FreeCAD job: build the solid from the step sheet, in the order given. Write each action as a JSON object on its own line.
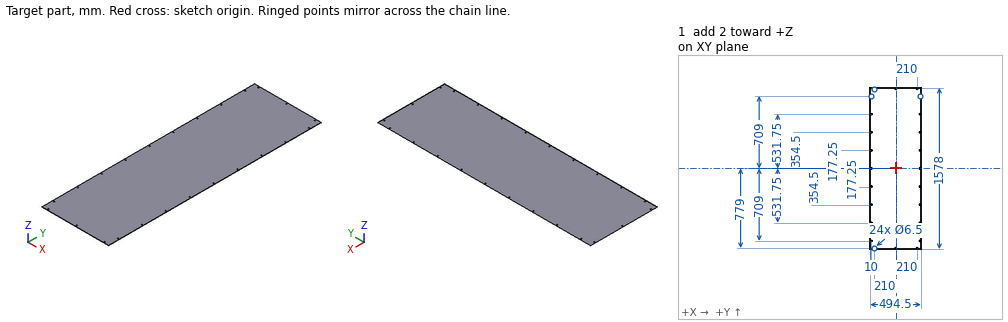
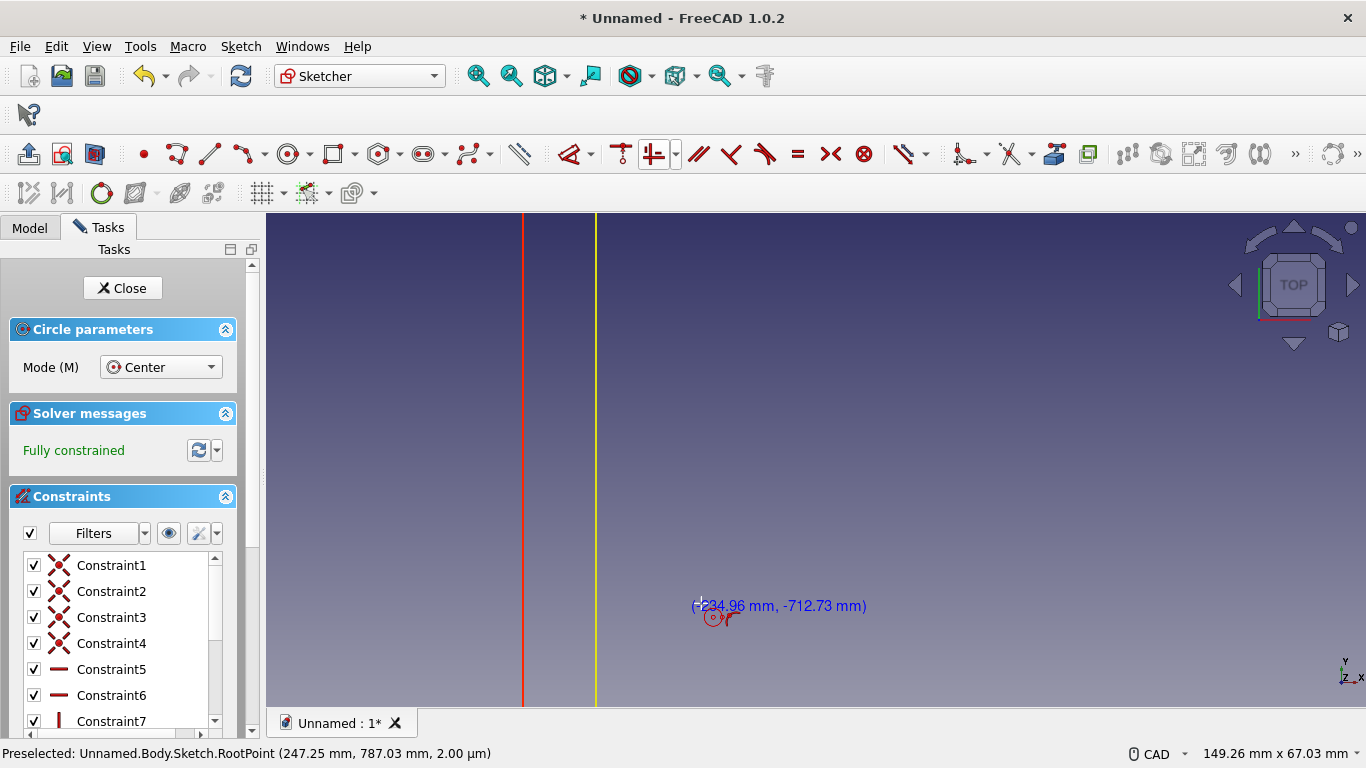
{"action": "scroll", "coordinate": [701, 603], "scroll_direction": "down", "scroll_amount": 18}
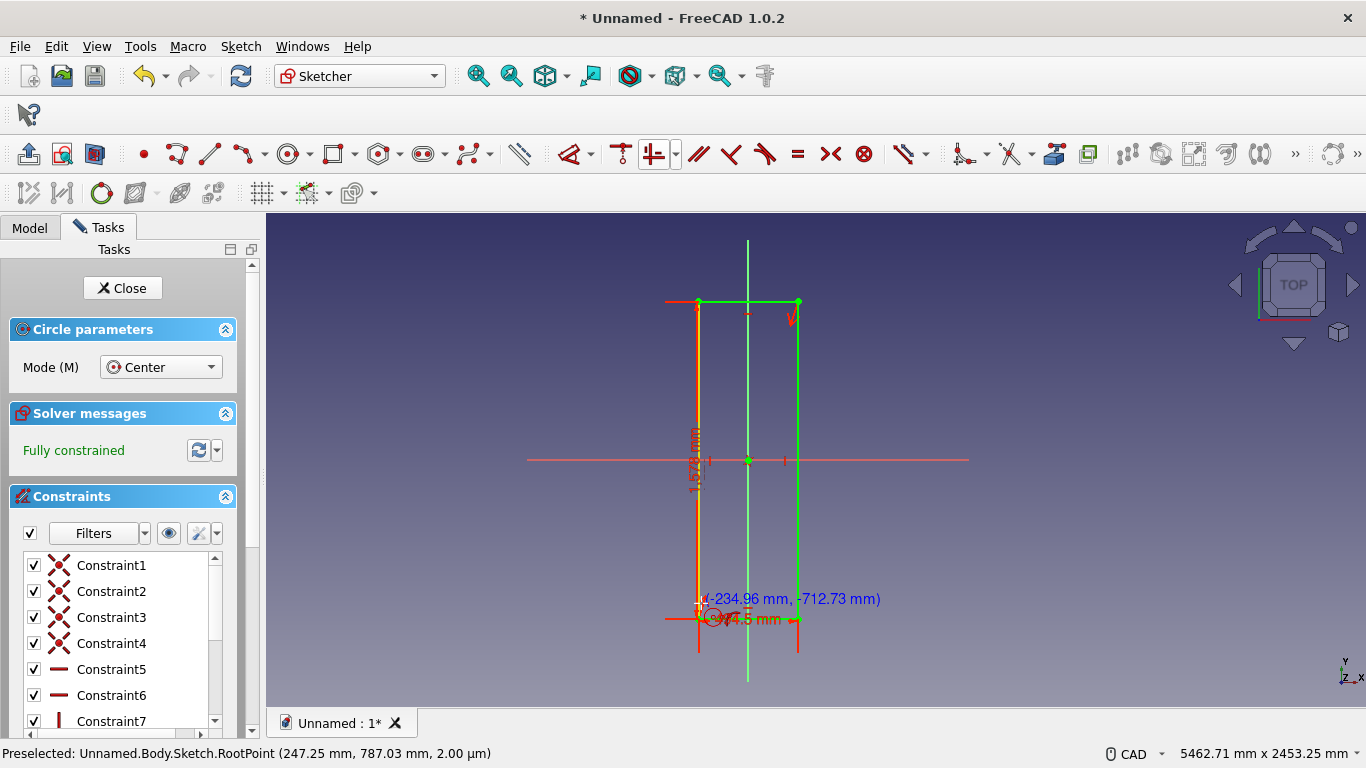
{"action": "scroll", "coordinate": [701, 603], "scroll_direction": "up", "scroll_amount": 11}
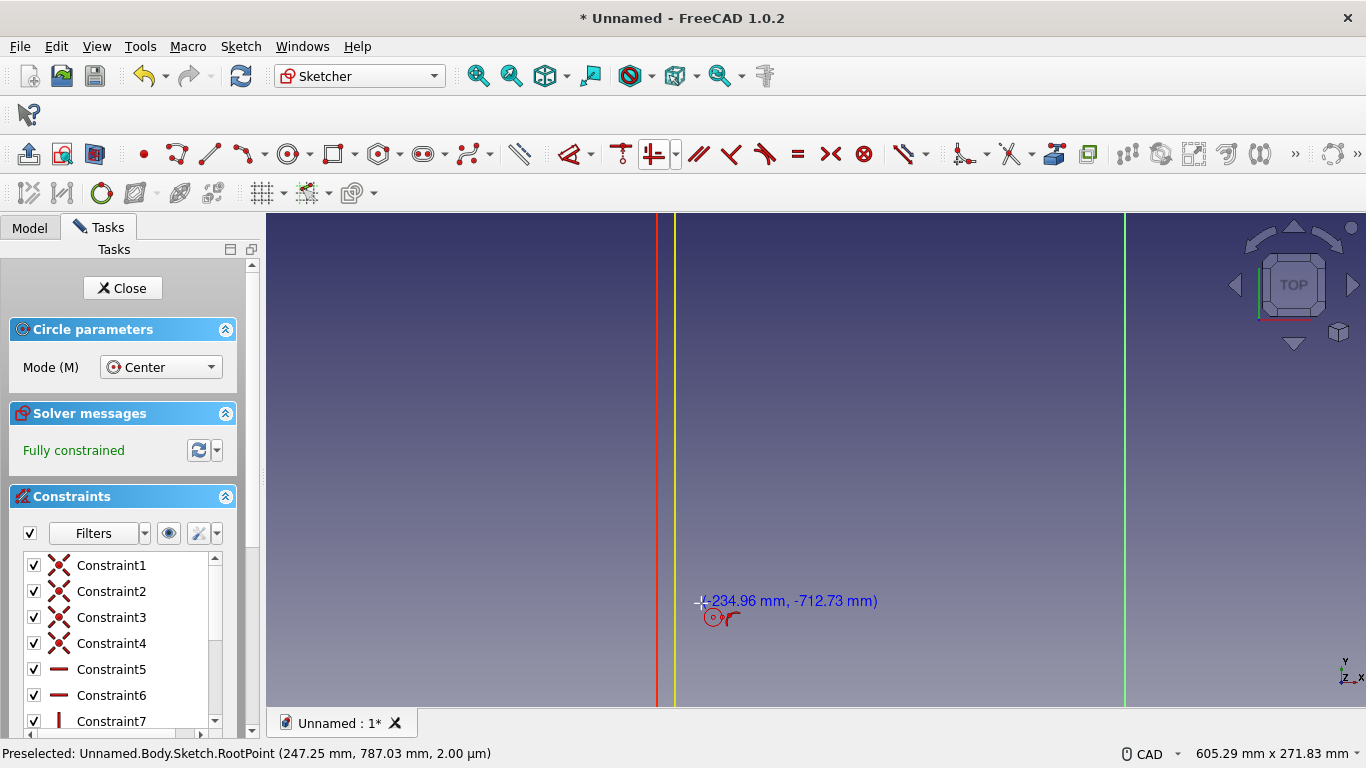
{"action": "left_click", "coordinate": [694, 599]}
{"action": "mouse_move", "coordinate": [698, 595]}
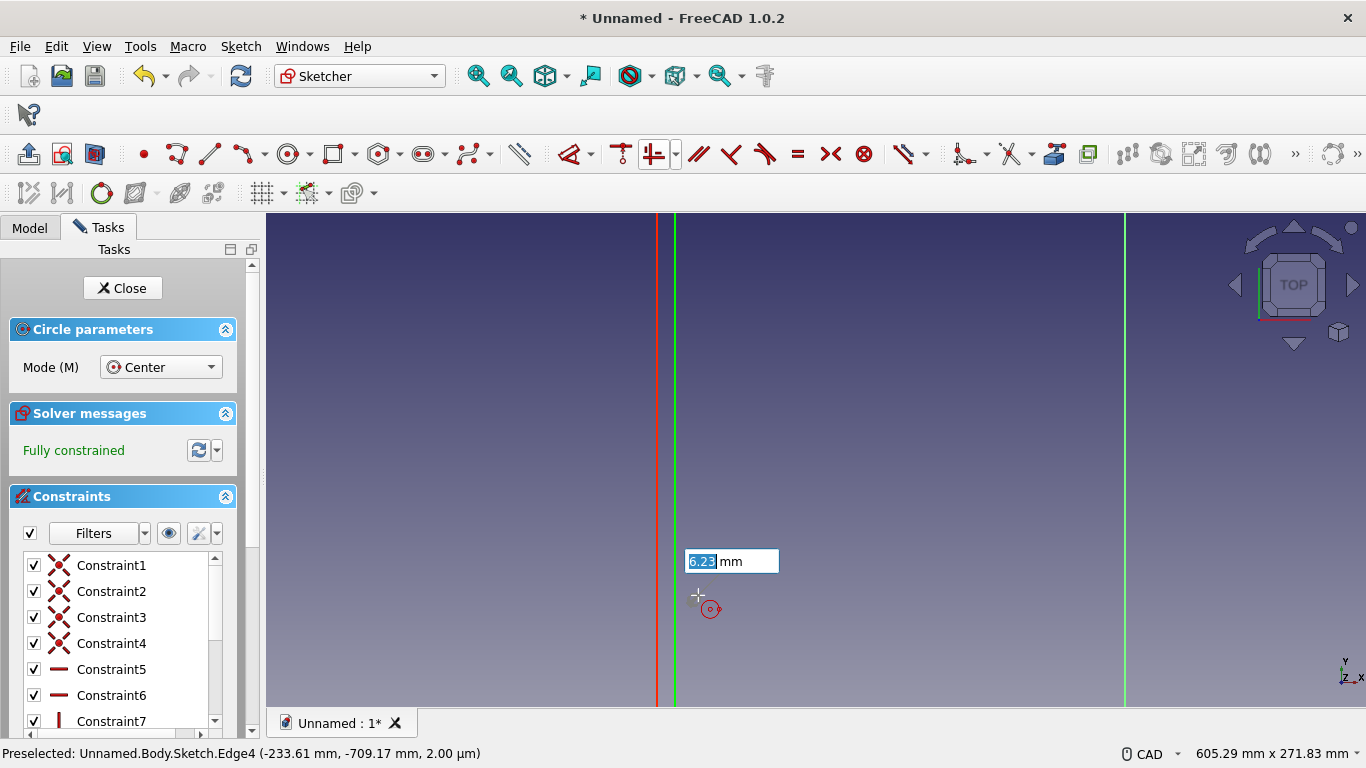
{"action": "type", "text": "6.5"}
{"action": "key", "text": "Return"}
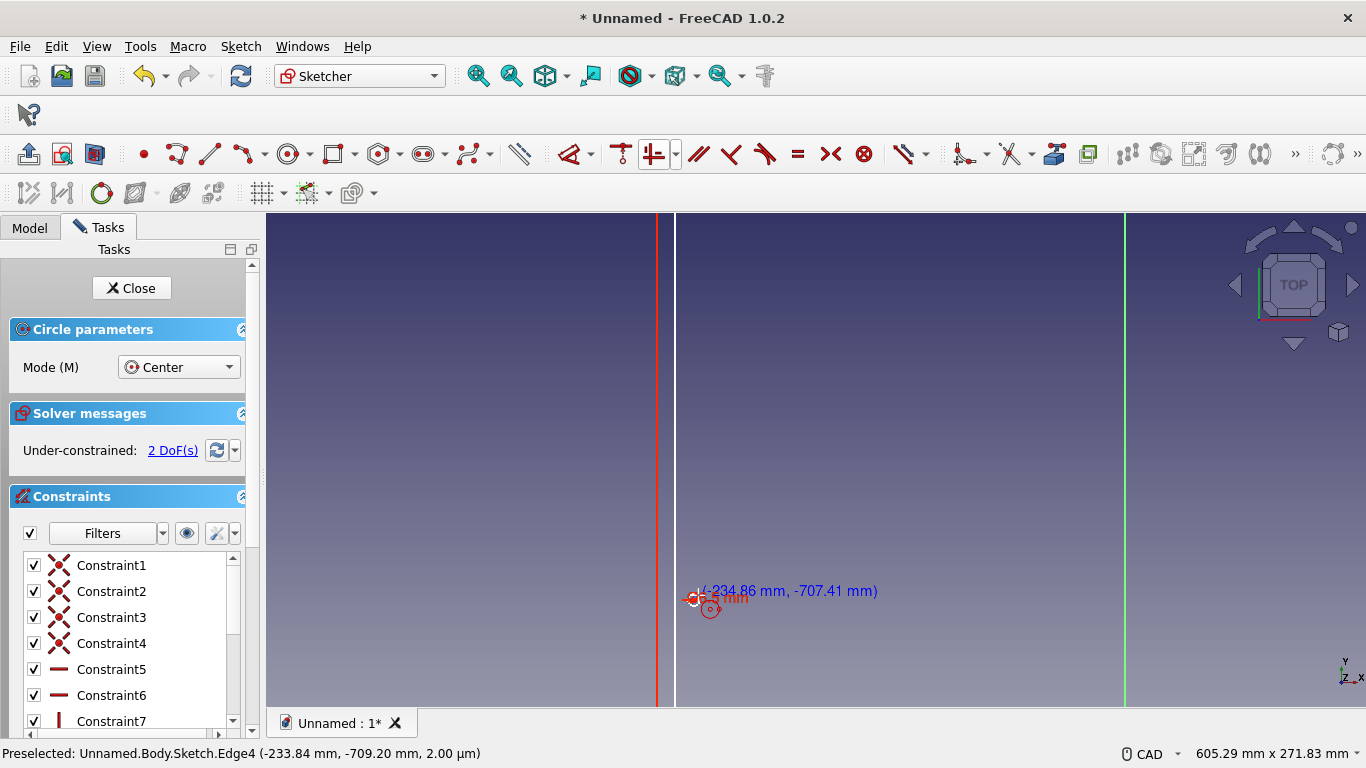
{"action": "scroll", "coordinate": [700, 603], "scroll_direction": "down", "scroll_amount": 11}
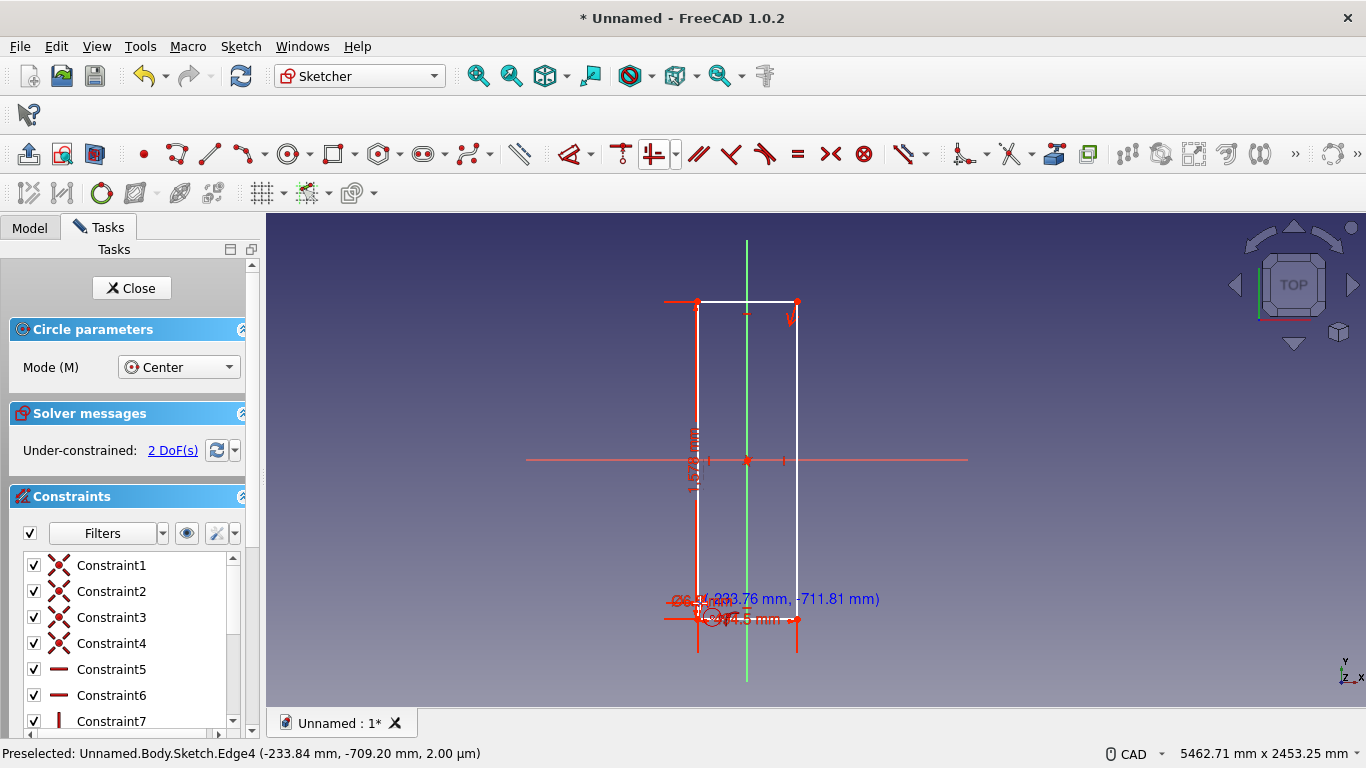
{"action": "scroll", "coordinate": [705, 617], "scroll_direction": "up", "scroll_amount": 18}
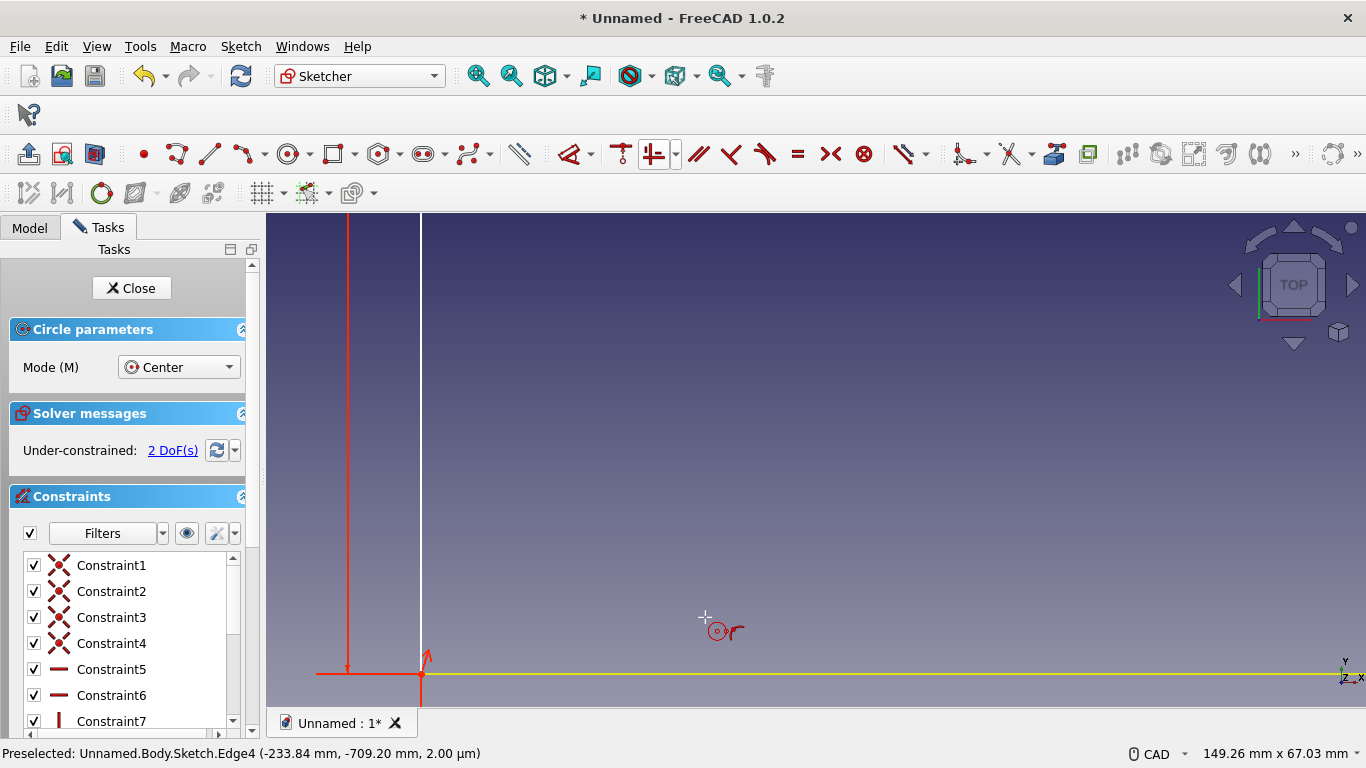
{"action": "scroll", "coordinate": [705, 617], "scroll_direction": "down", "scroll_amount": 18}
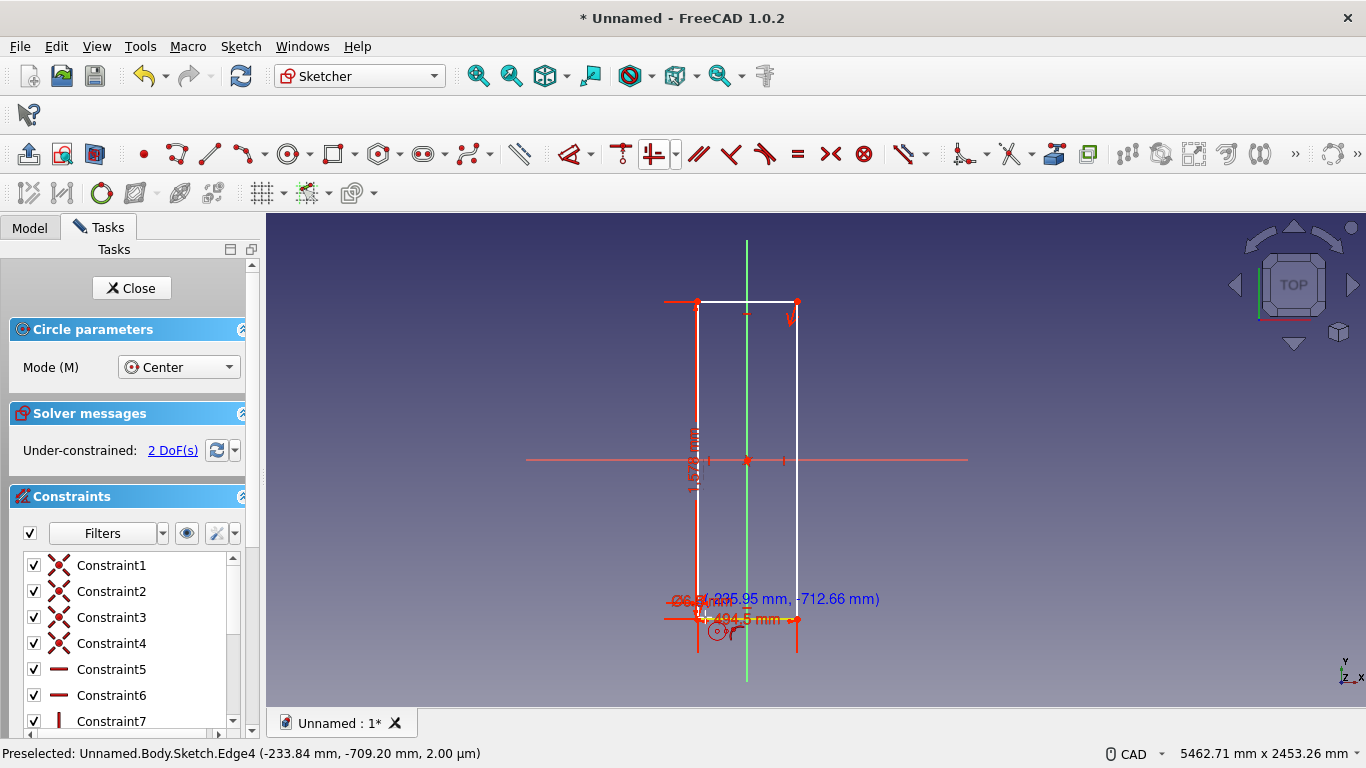
{"action": "scroll", "coordinate": [705, 617], "scroll_direction": "up", "scroll_amount": 11}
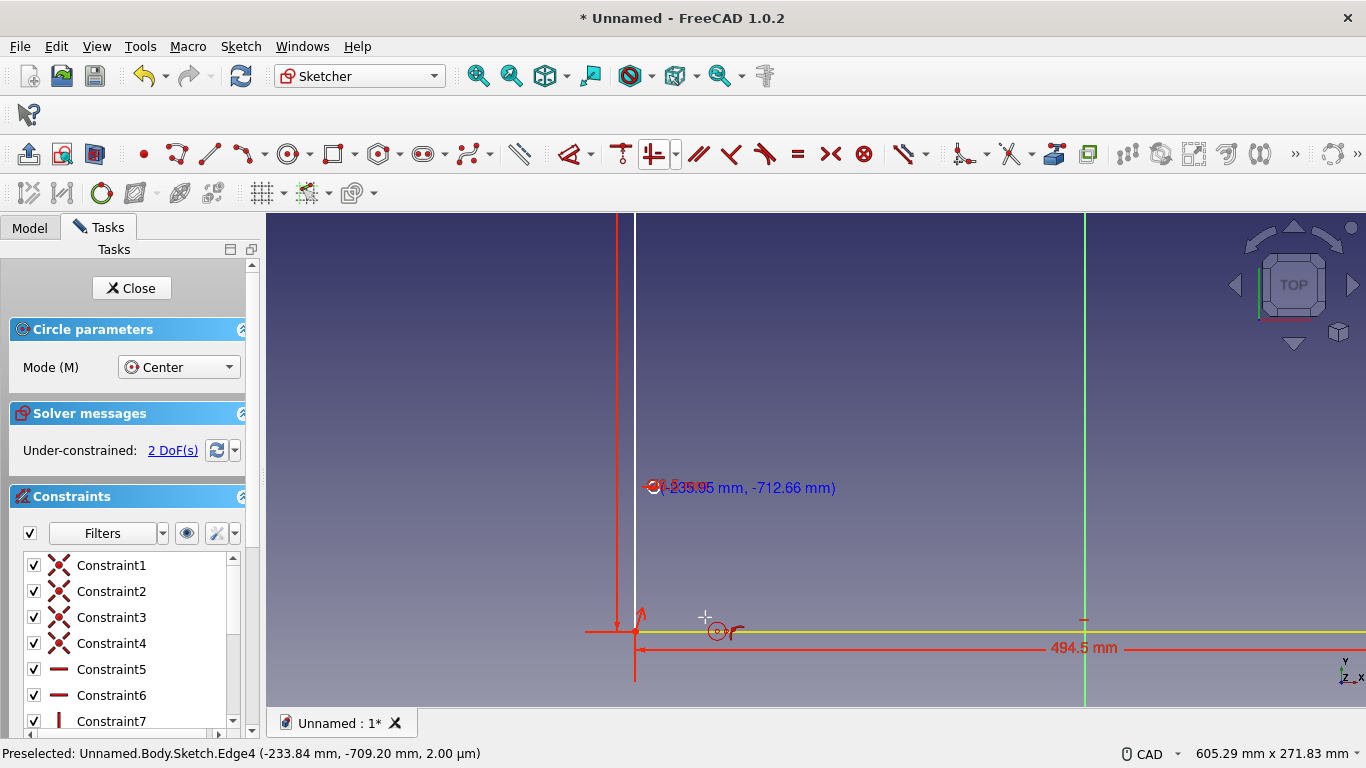
{"action": "left_click", "coordinate": [703, 614]}
{"action": "mouse_move", "coordinate": [707, 609]}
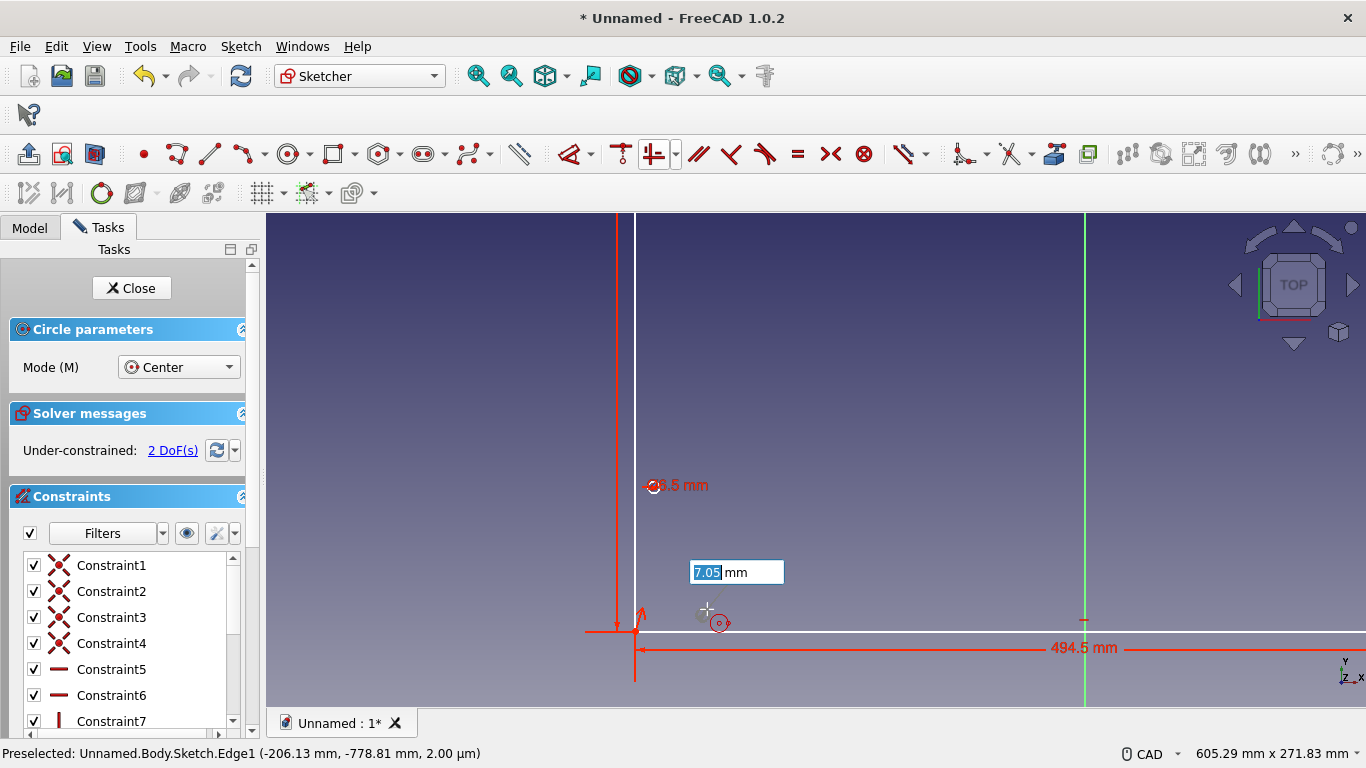
{"action": "type", "text": "6.5"}
{"action": "key", "text": "Return"}